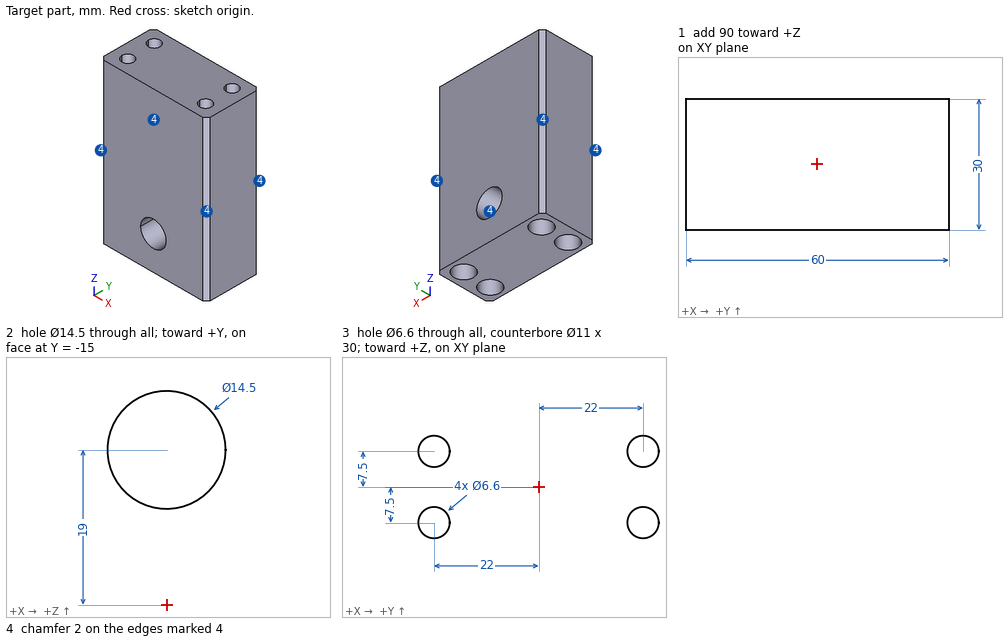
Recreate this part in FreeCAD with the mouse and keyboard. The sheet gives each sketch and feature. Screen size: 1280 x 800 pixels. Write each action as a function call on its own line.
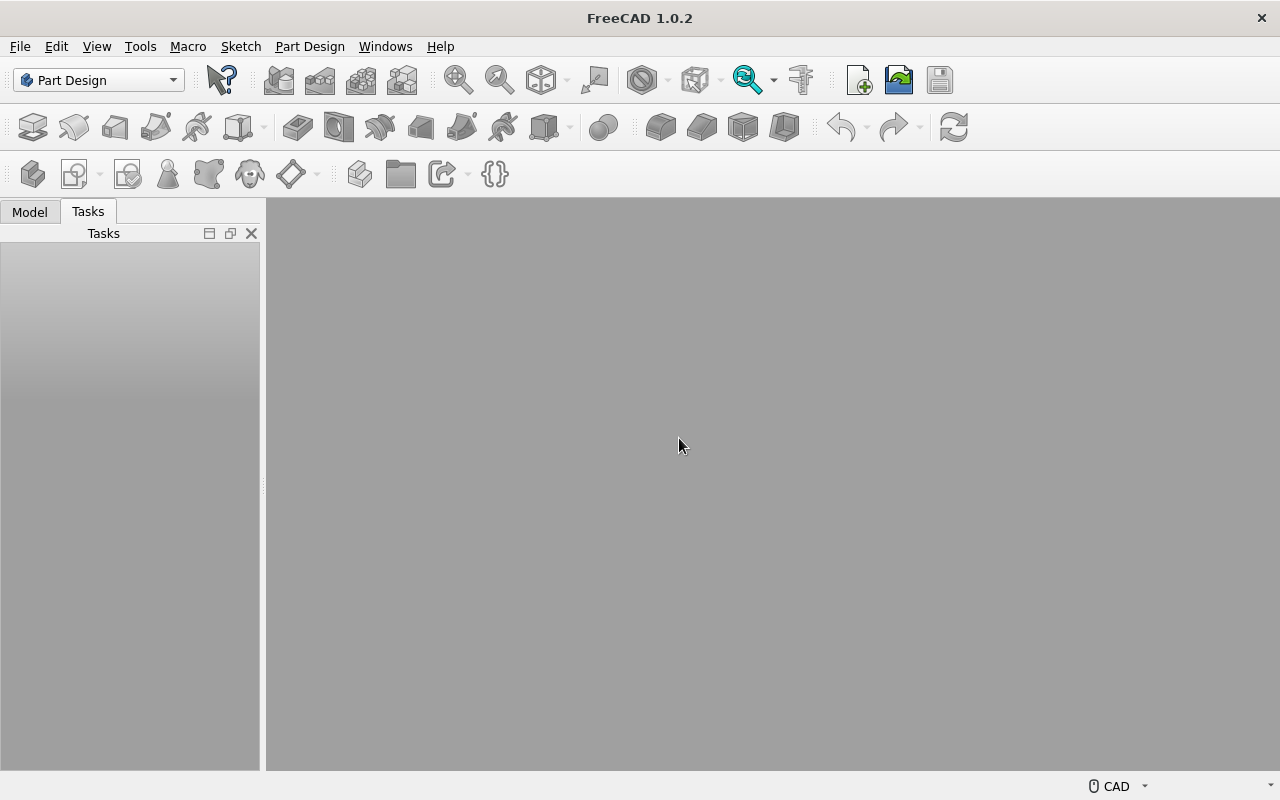
key(ctrl+n)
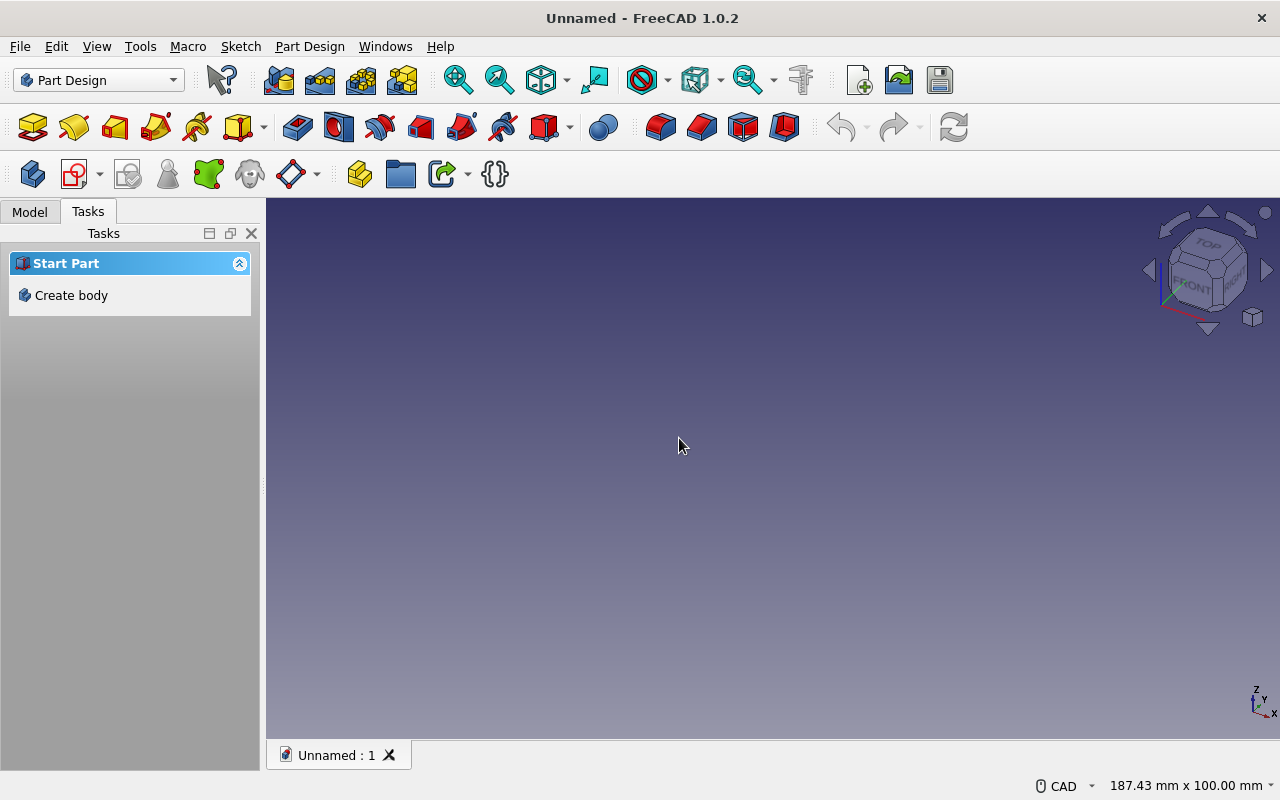
click(74, 174)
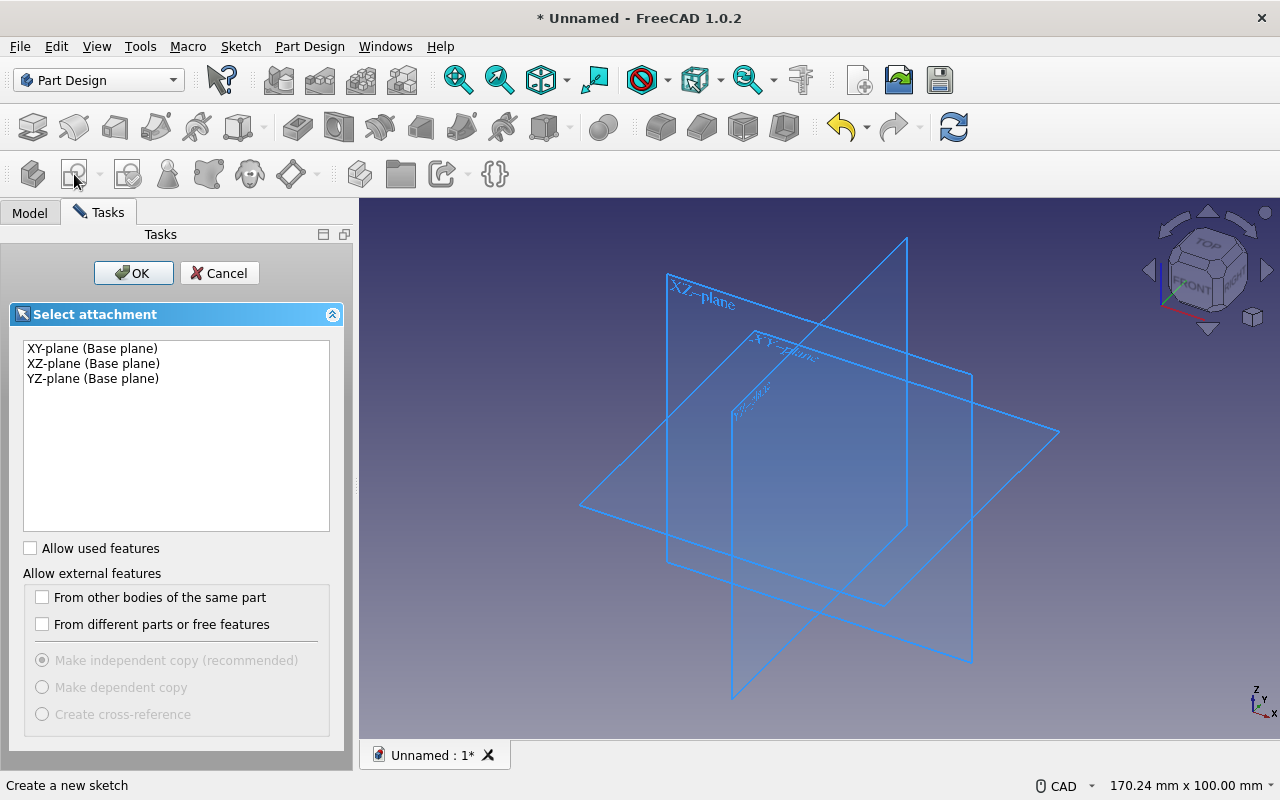
click(84, 348)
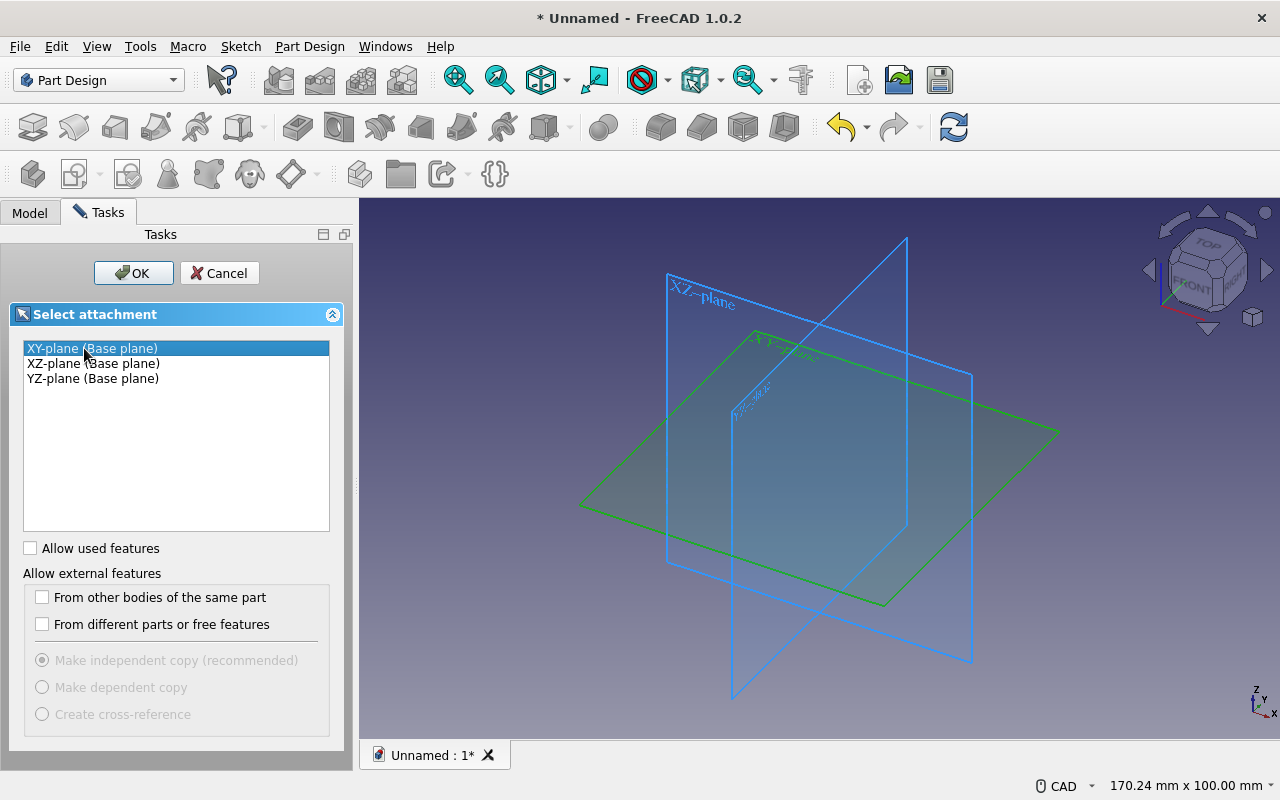
click(134, 273)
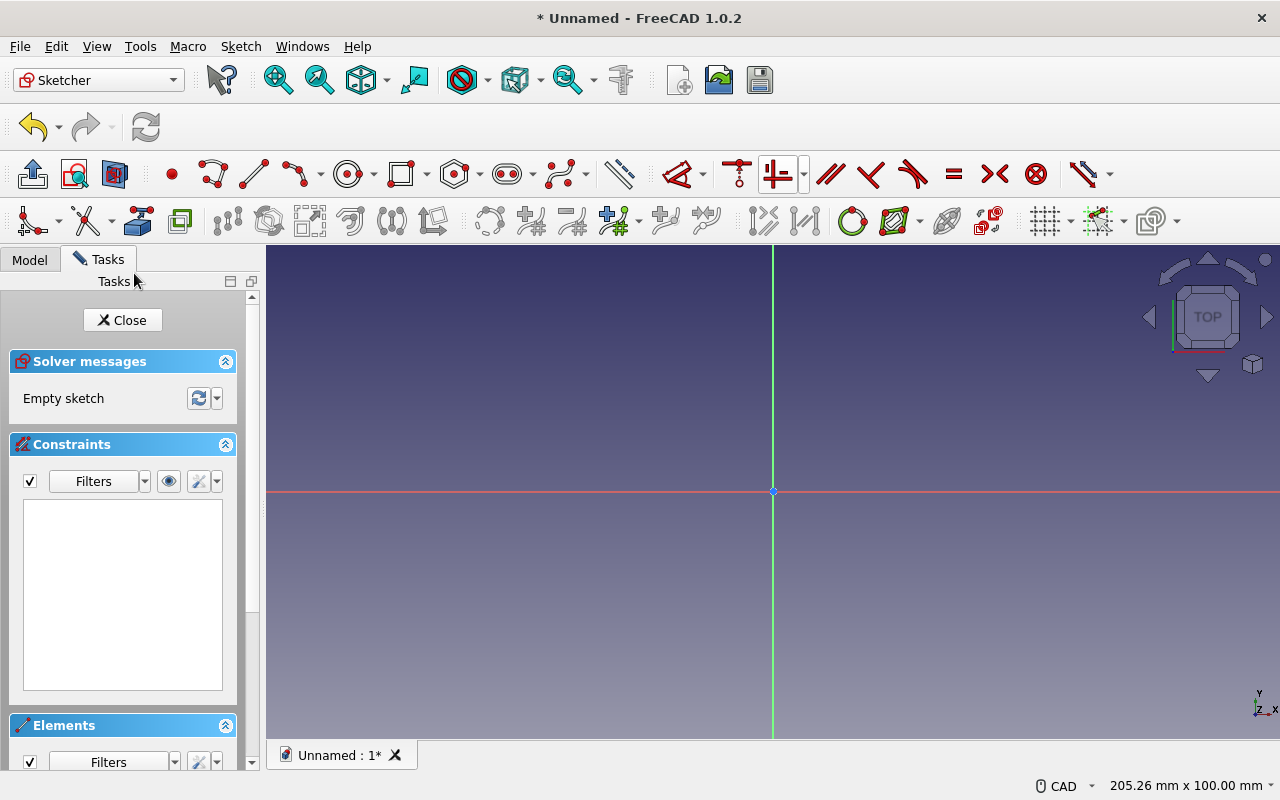
scroll(856, 492, up, 3)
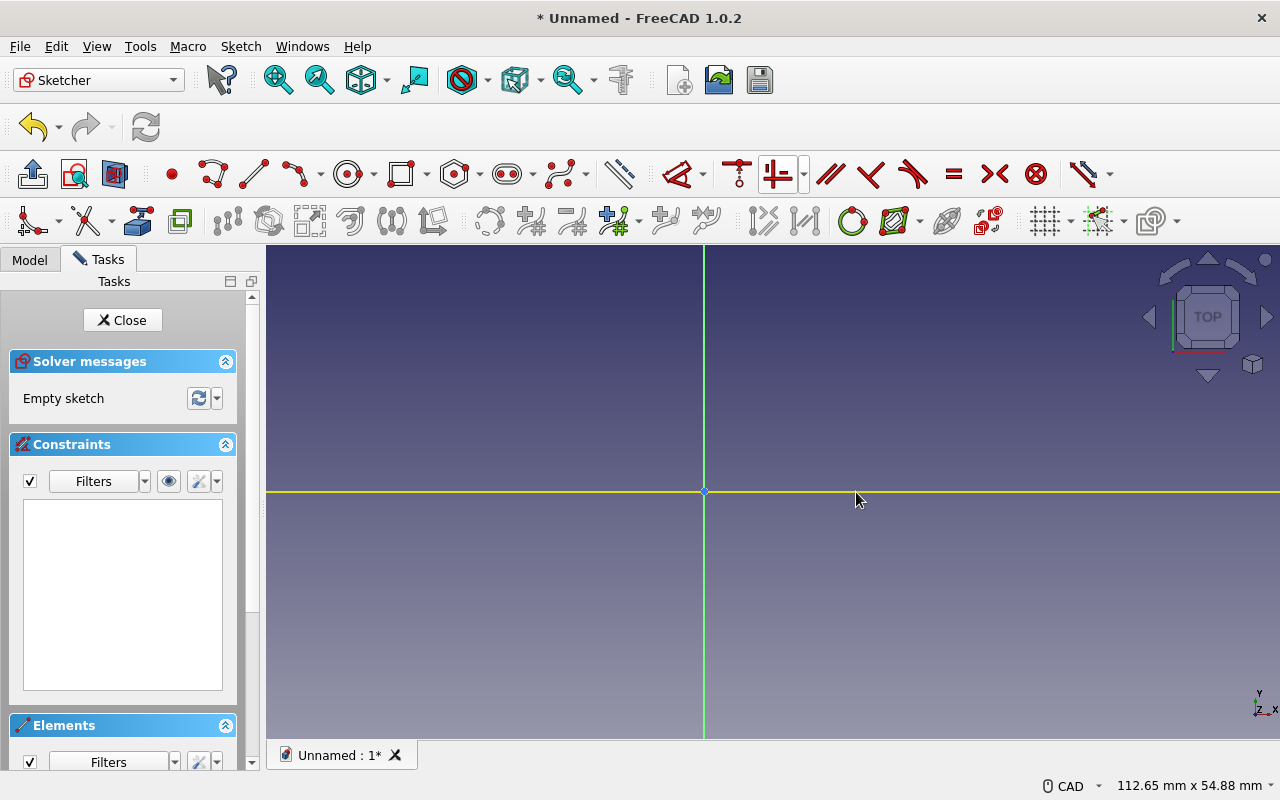
key(g)
key(v)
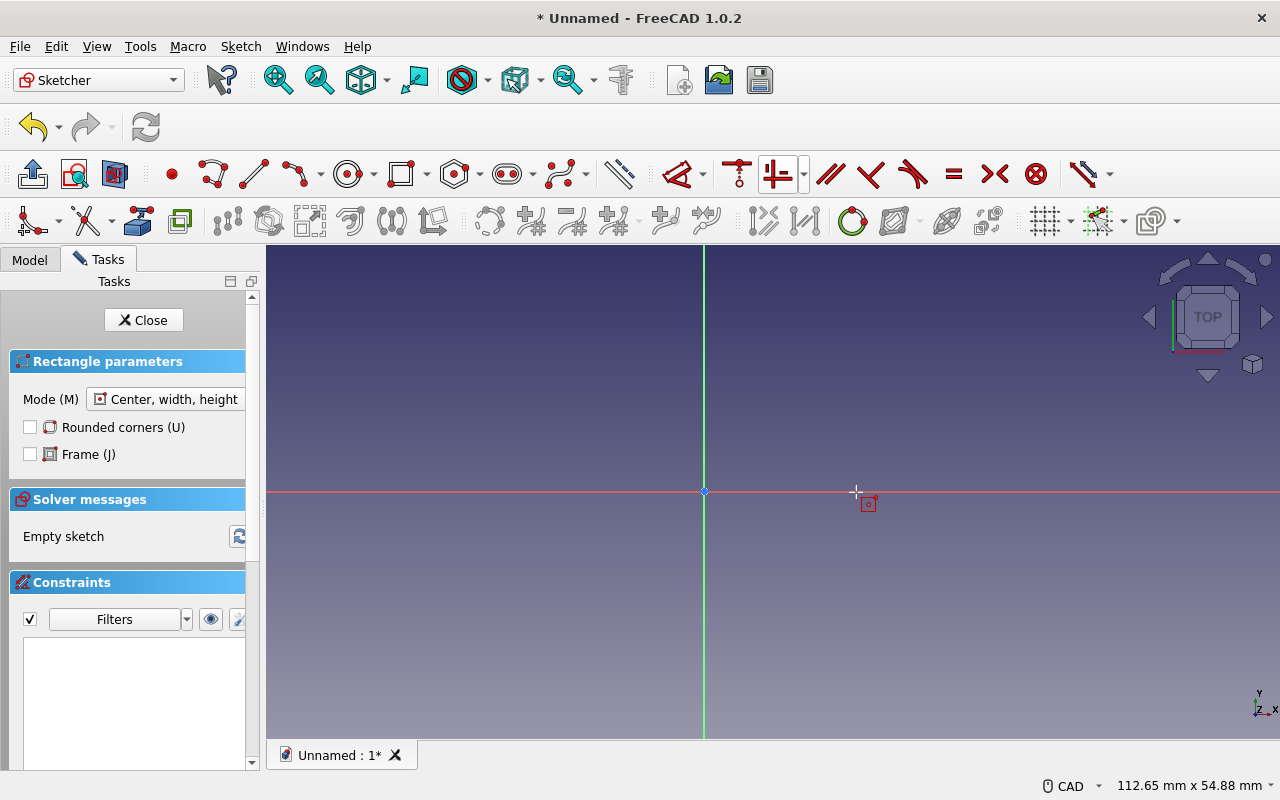
click(704, 492)
click(974, 357)
key(Escape)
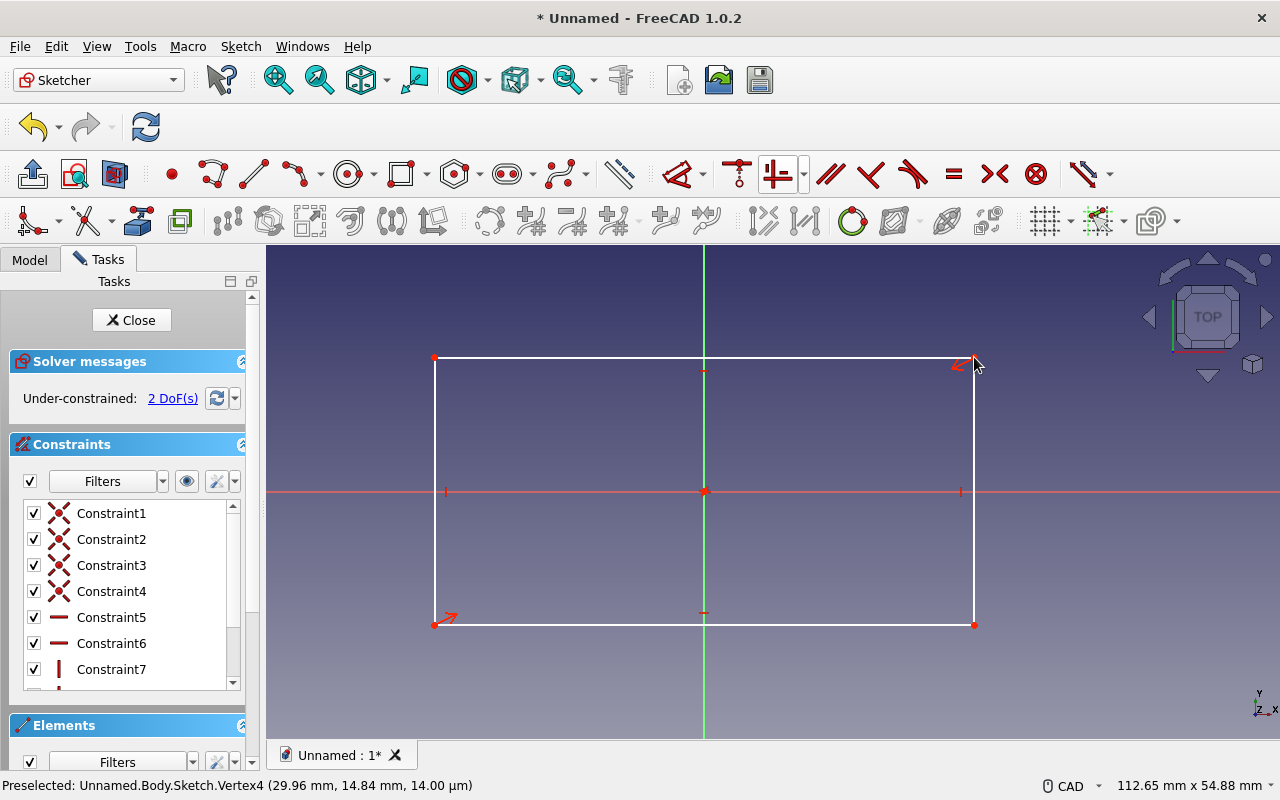
click(676, 174)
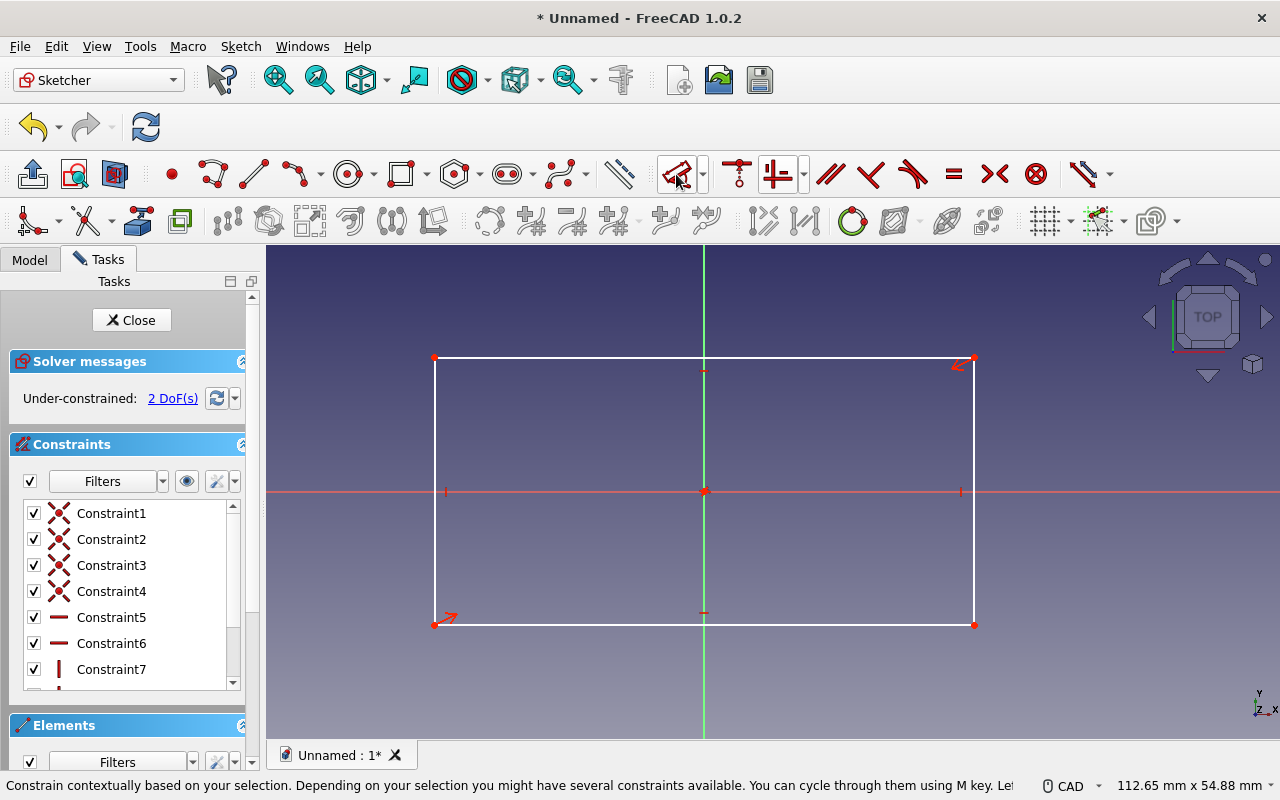
click(596, 625)
click(580, 659)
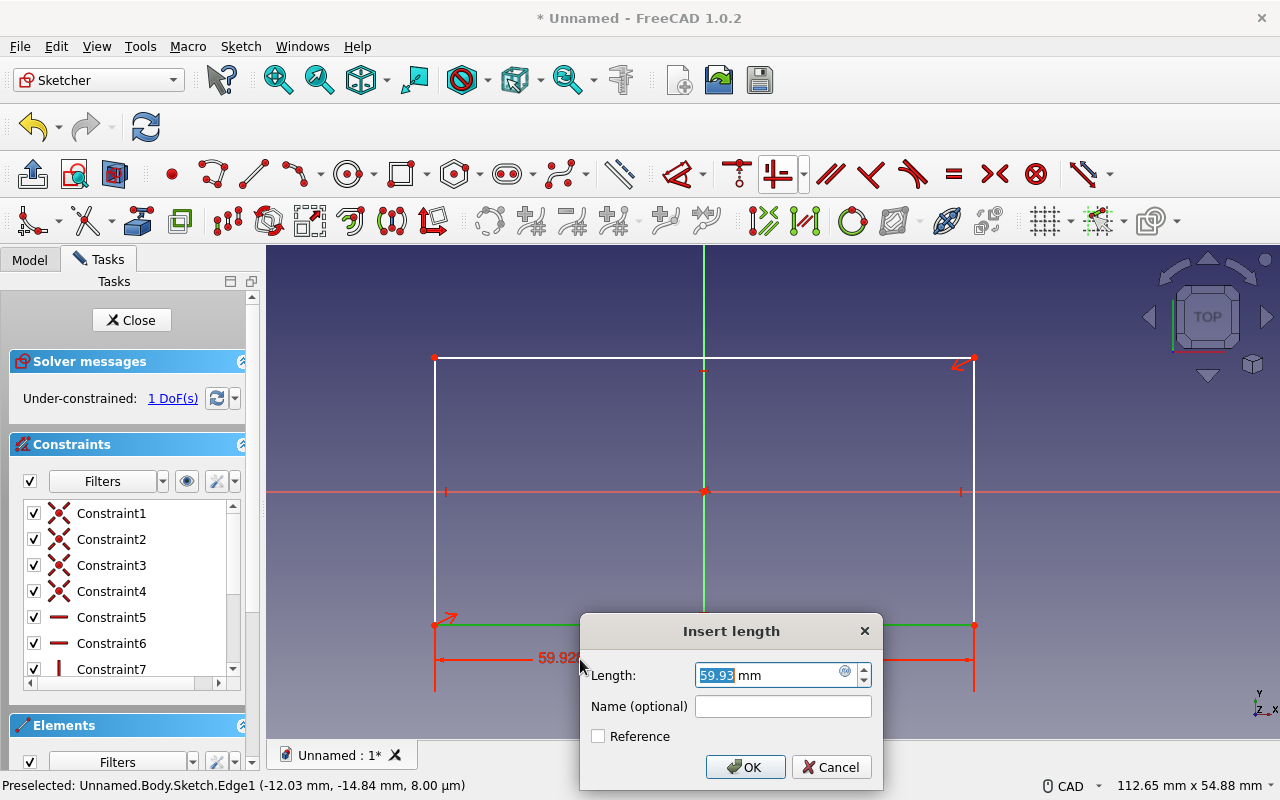
text(60)
key(Return)